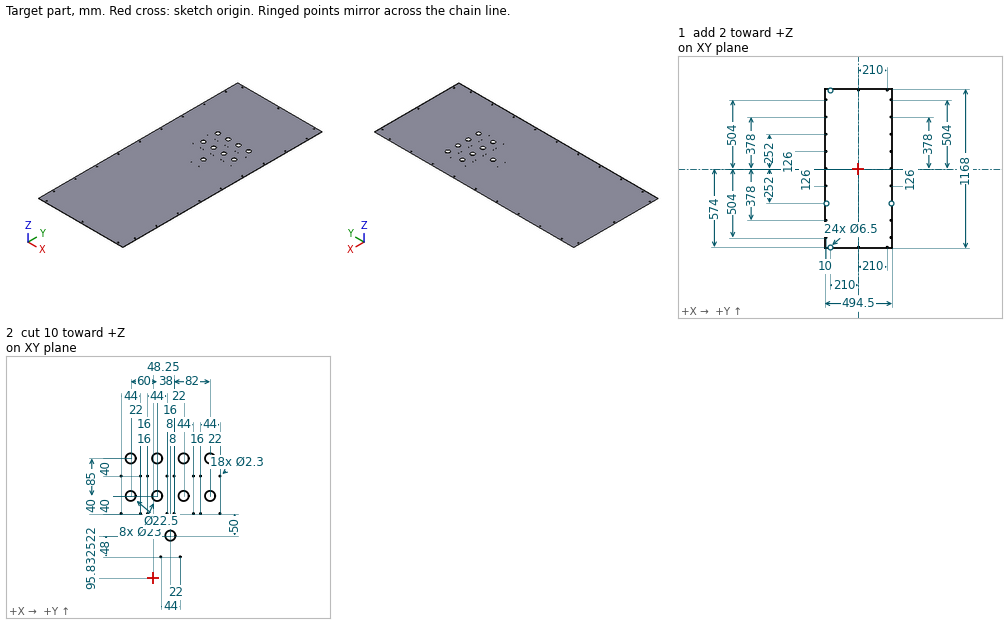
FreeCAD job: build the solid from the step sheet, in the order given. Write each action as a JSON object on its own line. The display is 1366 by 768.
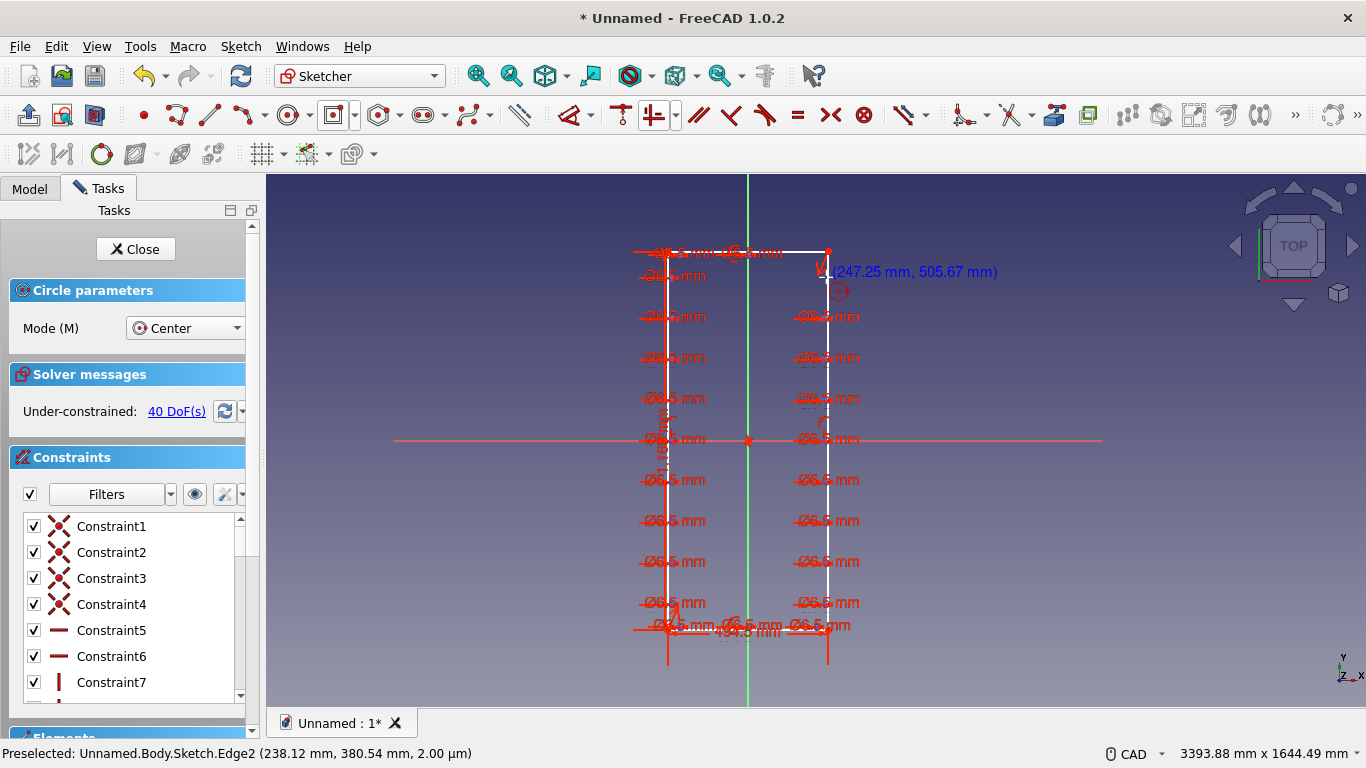
{"action": "scroll", "coordinate": [825, 278], "scroll_direction": "up", "scroll_amount": 8}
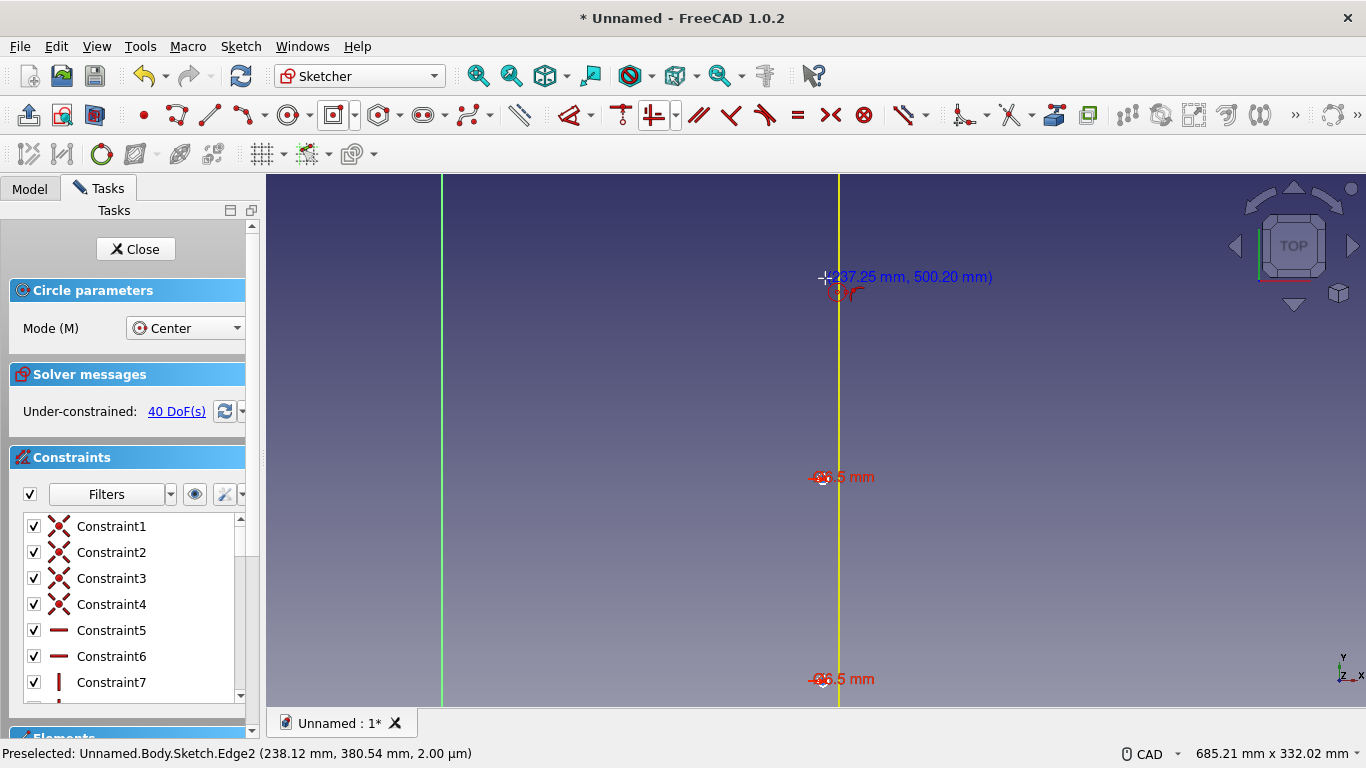
{"action": "left_click", "coordinate": [823, 276]}
{"action": "mouse_move", "coordinate": [819, 272]}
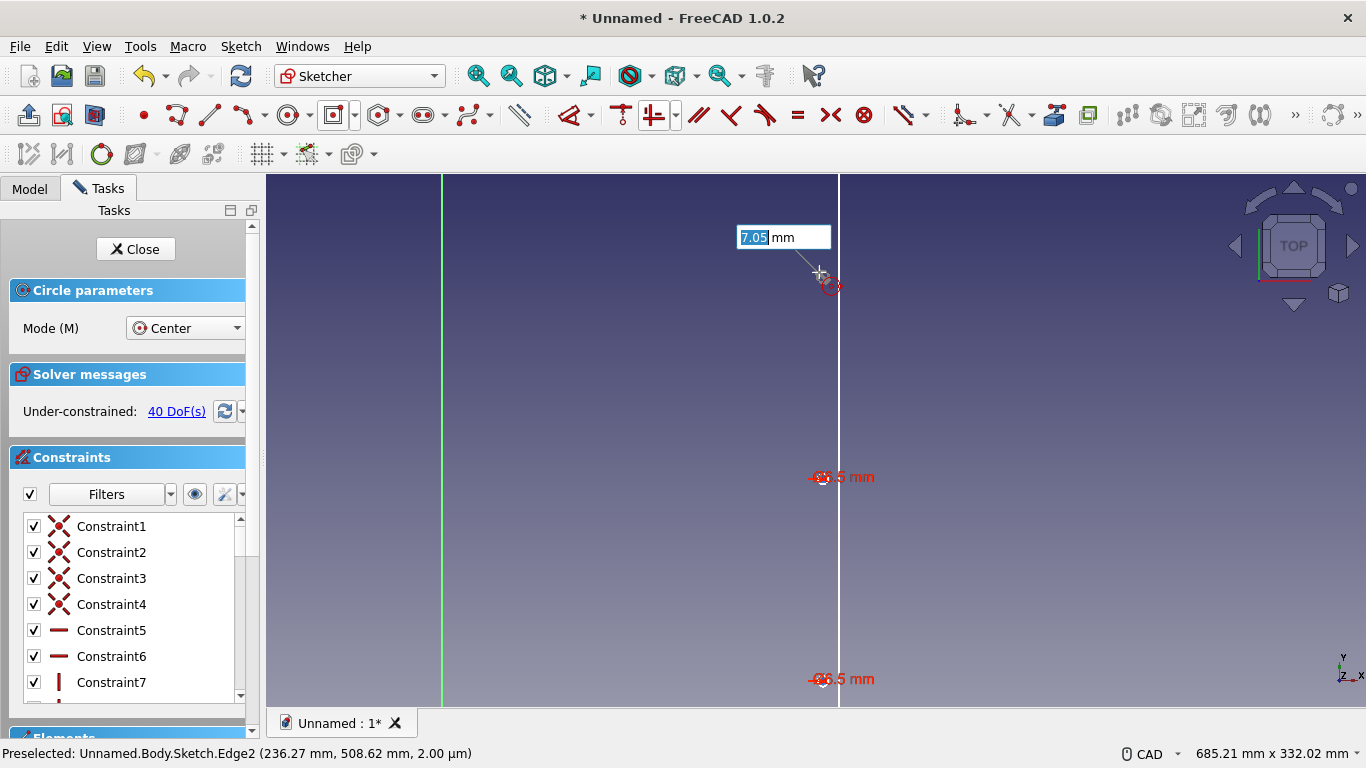
{"action": "type", "text": "6.5"}
{"action": "key", "text": "Return"}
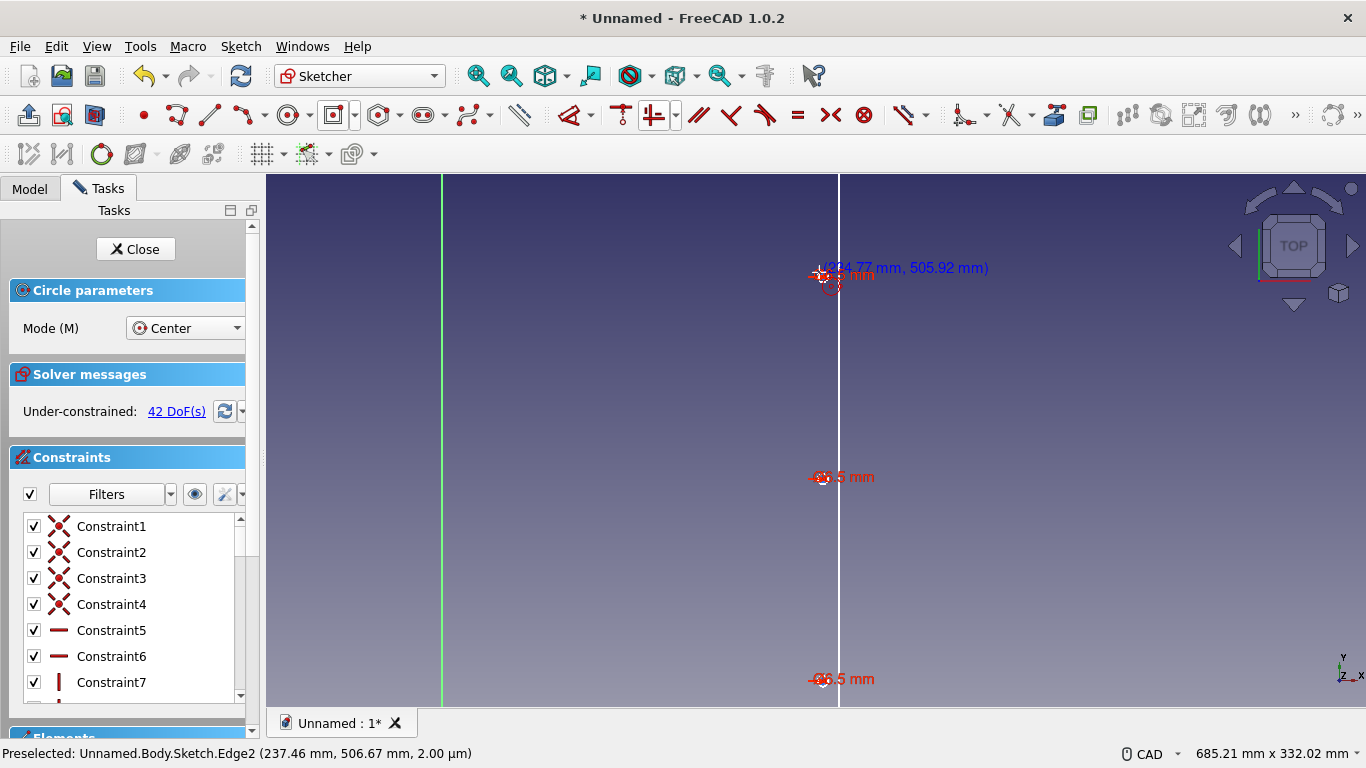
{"action": "scroll", "coordinate": [808, 313], "scroll_direction": "down", "scroll_amount": 9}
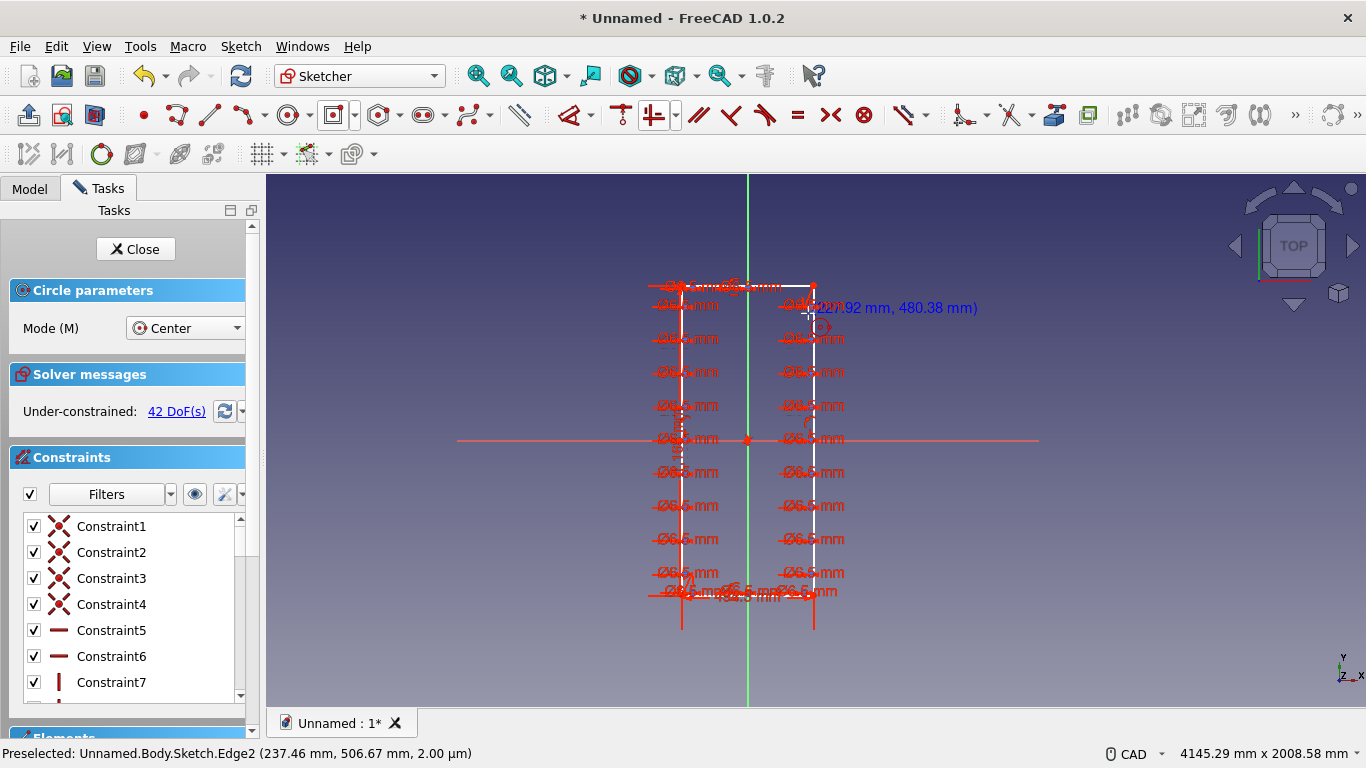
{"action": "scroll", "coordinate": [804, 289], "scroll_direction": "up", "scroll_amount": 17}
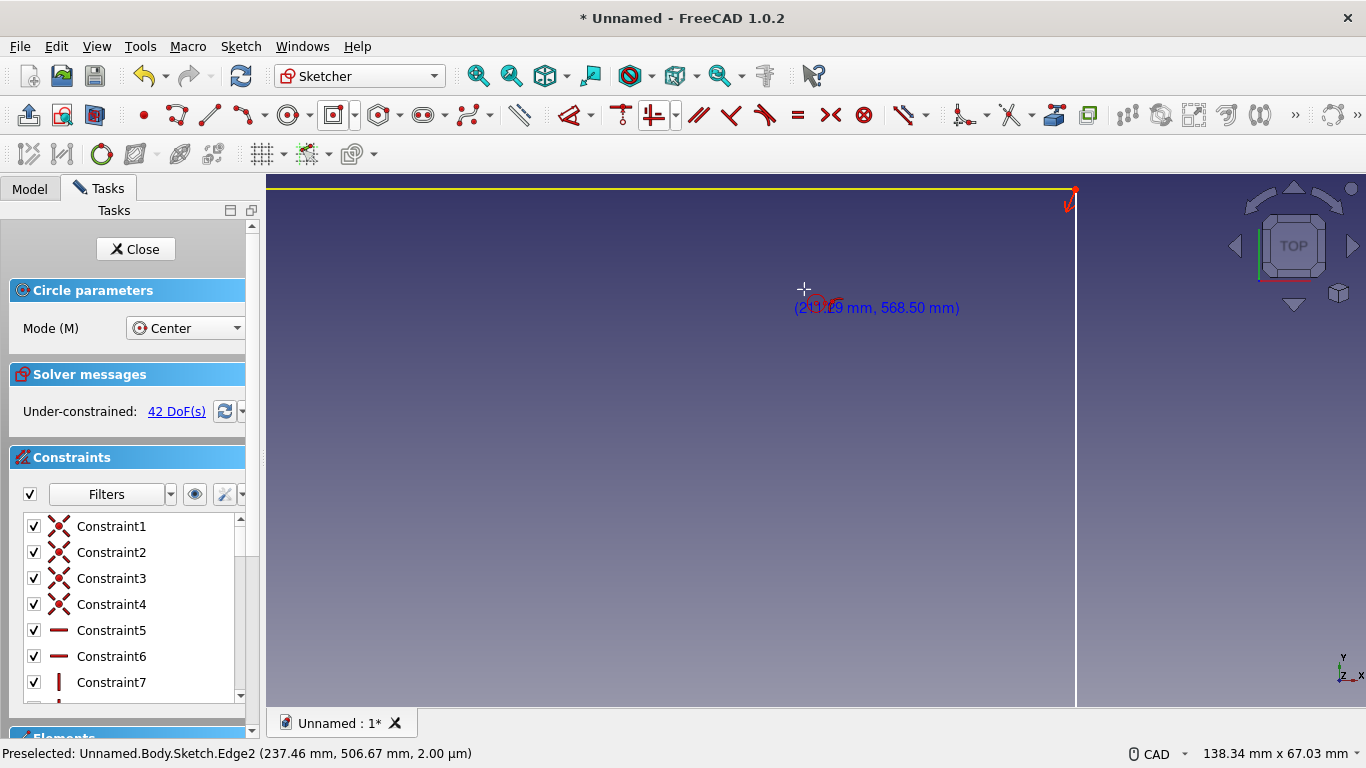
{"action": "scroll", "coordinate": [817, 254], "scroll_direction": "down", "scroll_amount": 16}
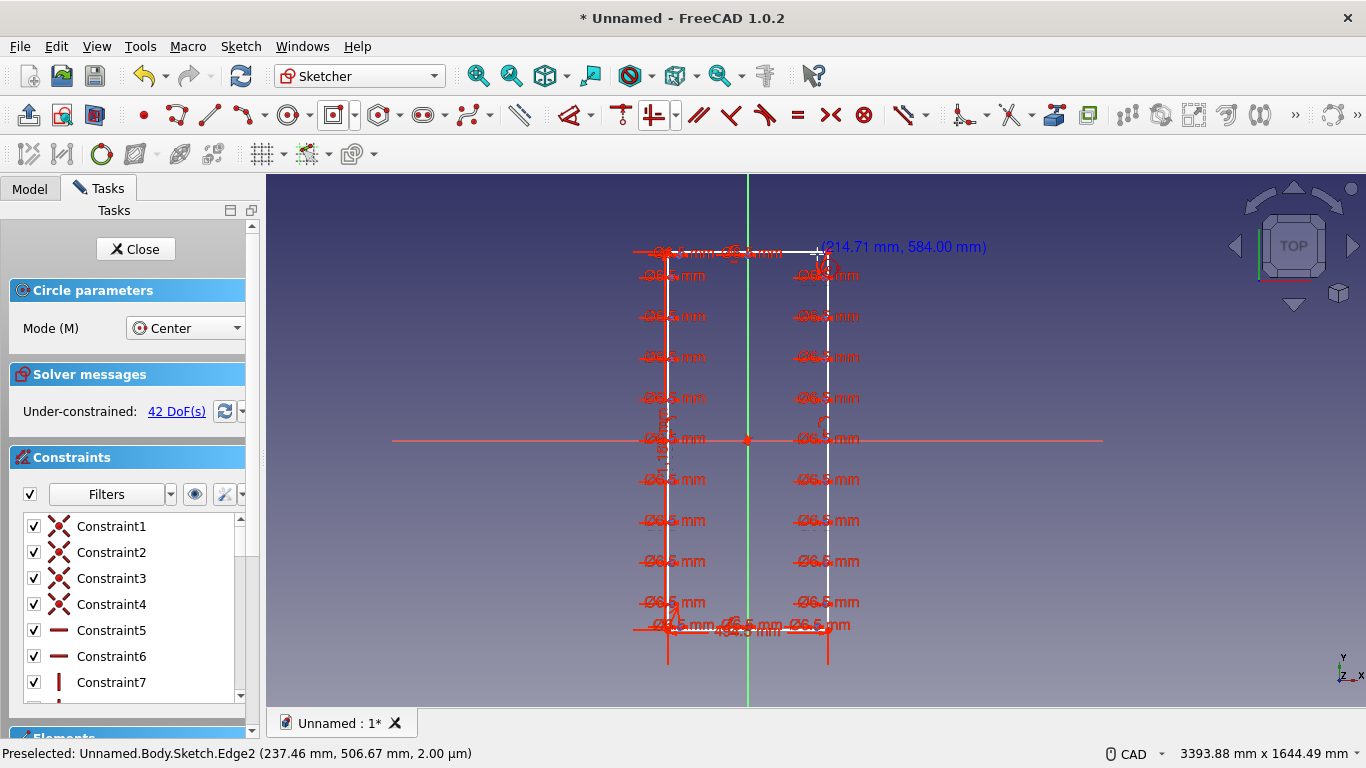
{"action": "scroll", "coordinate": [816, 255], "scroll_direction": "up", "scroll_amount": 8}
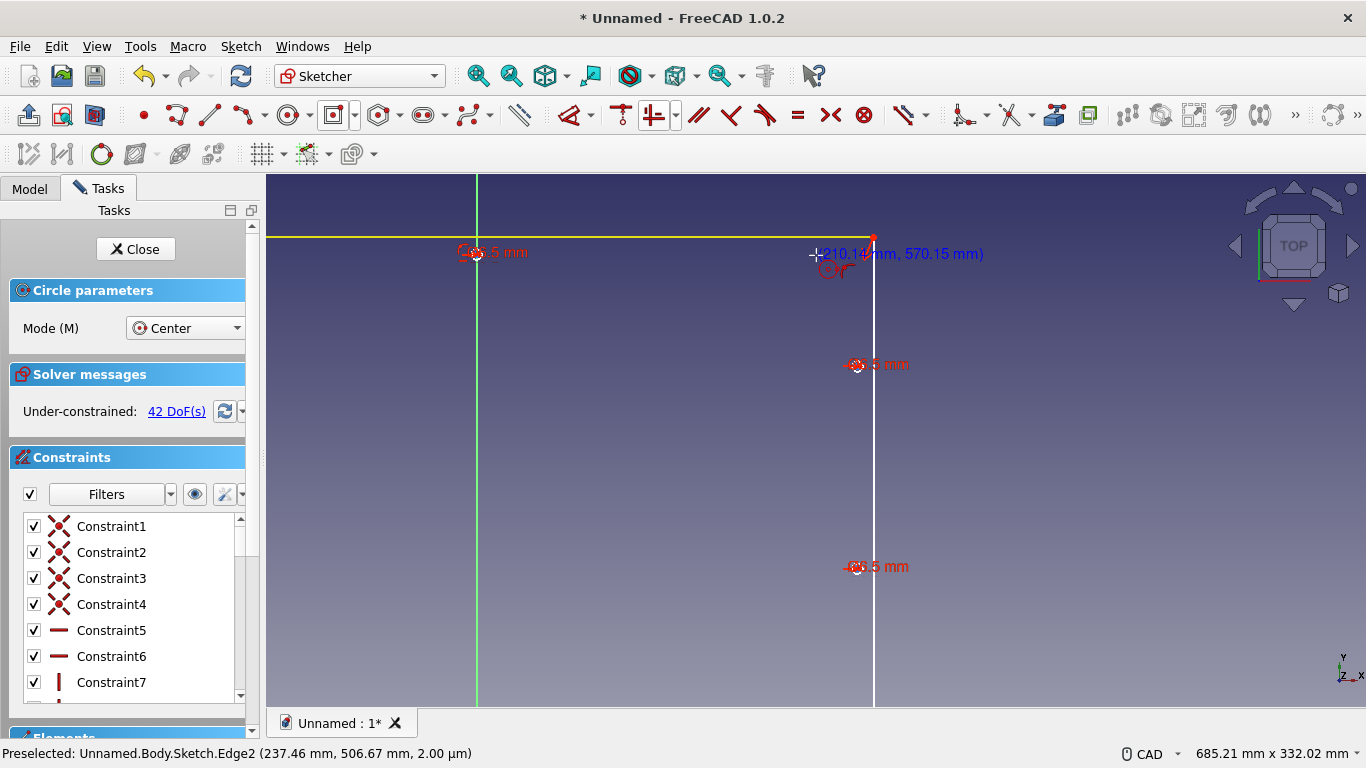
{"action": "left_click", "coordinate": [814, 253]}
{"action": "mouse_move", "coordinate": [817, 257]}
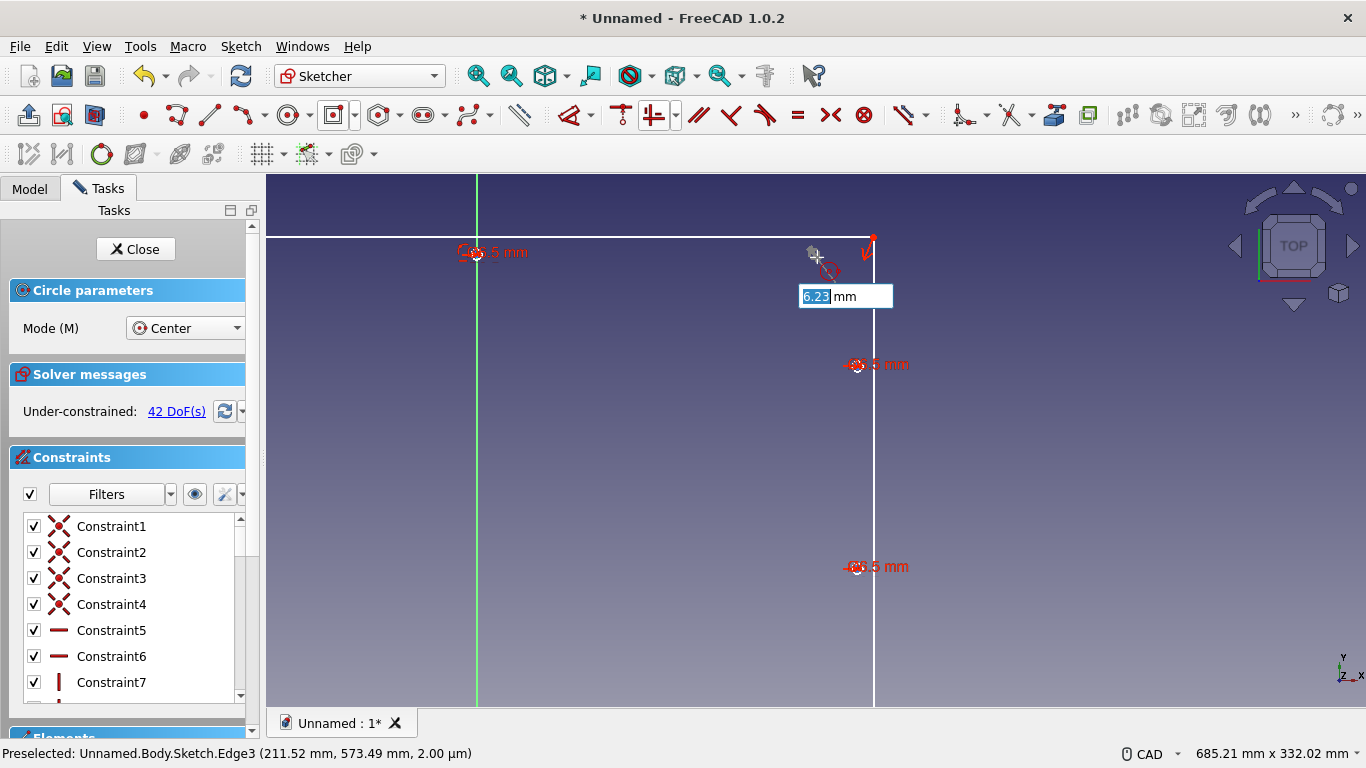
{"action": "type", "text": "6.5"}
{"action": "key", "text": "Return"}
{"action": "key", "text": "Escape"}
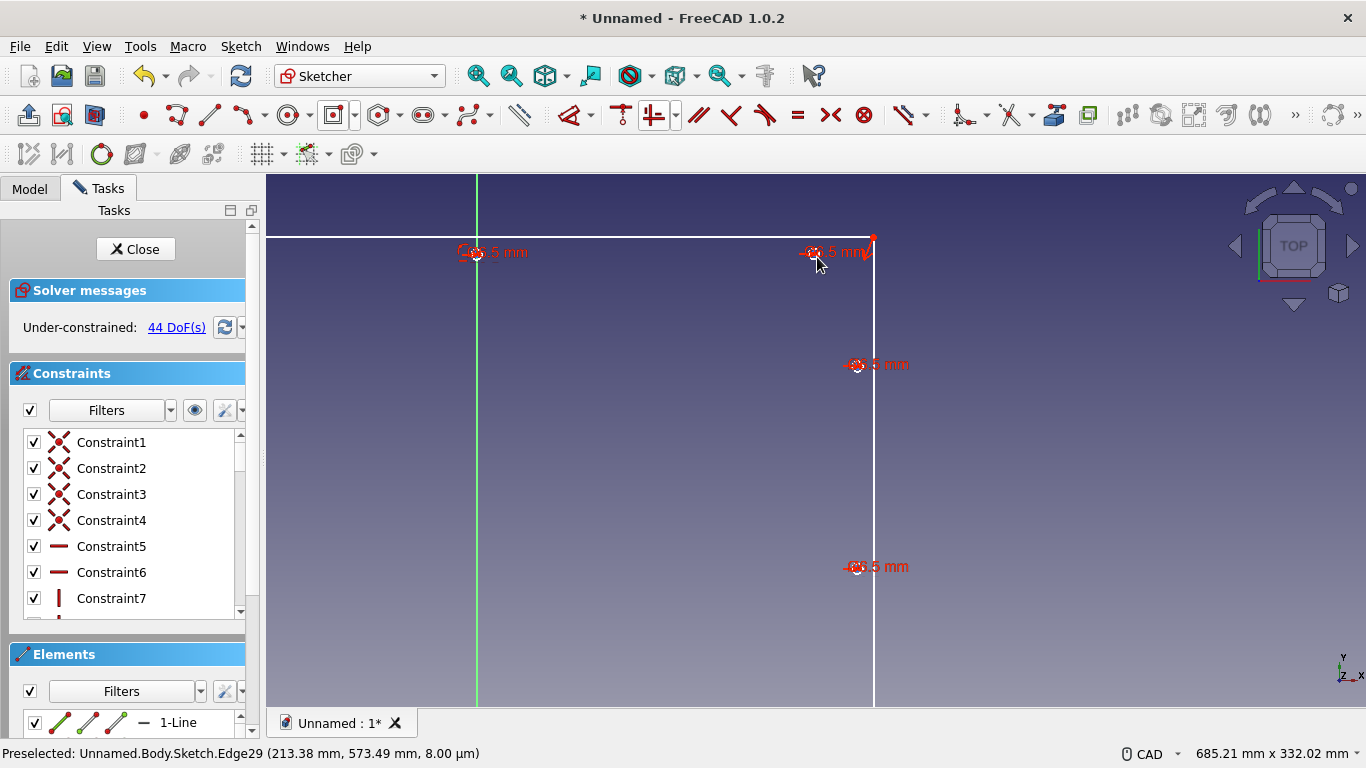
{"action": "scroll", "coordinate": [801, 295], "scroll_direction": "down", "scroll_amount": 9}